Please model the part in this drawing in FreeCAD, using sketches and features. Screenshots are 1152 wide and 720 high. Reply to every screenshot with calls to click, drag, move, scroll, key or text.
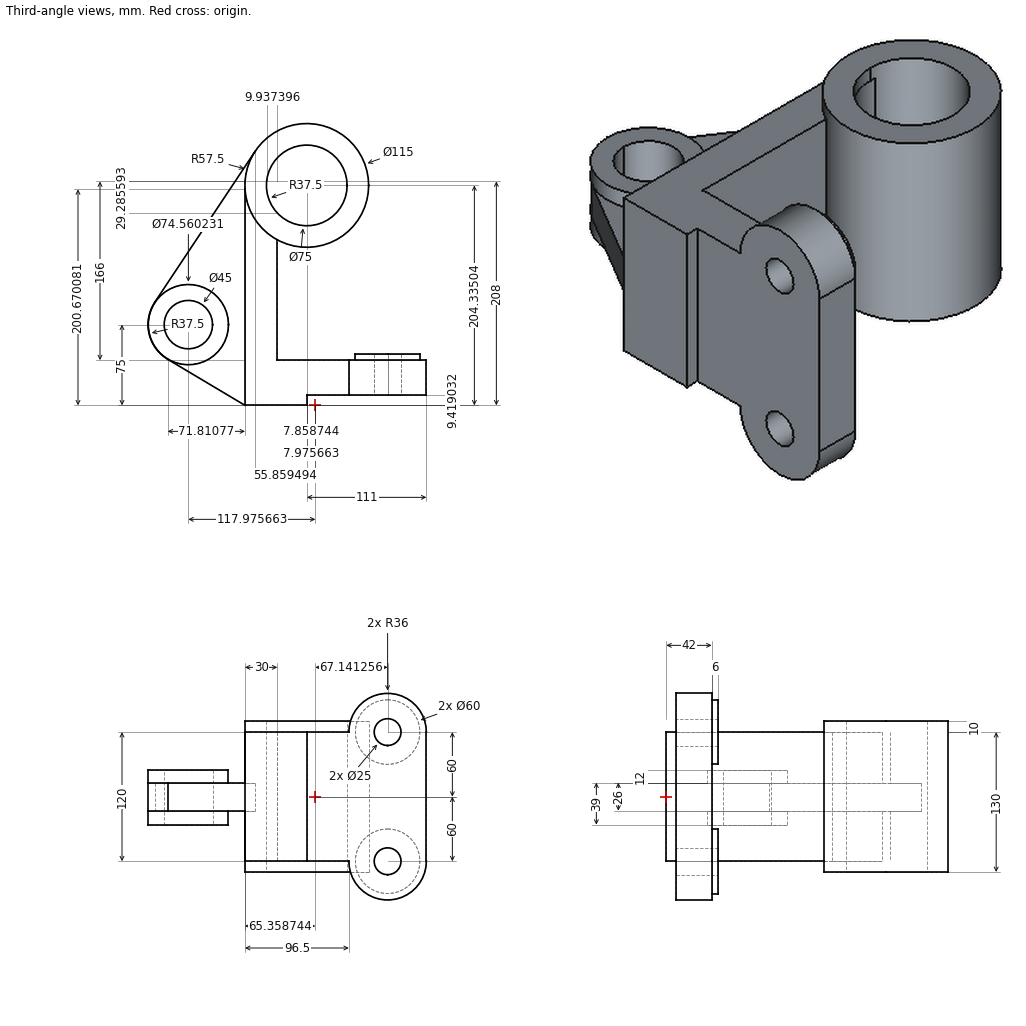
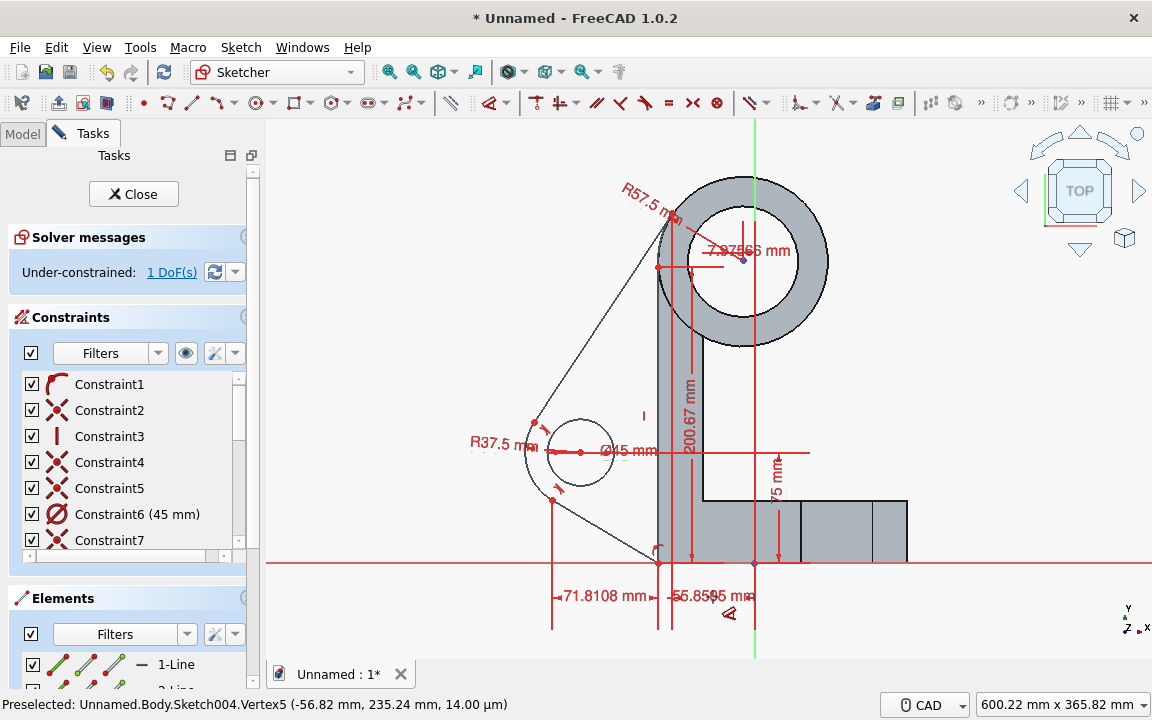
click(743, 261)
click(789, 412)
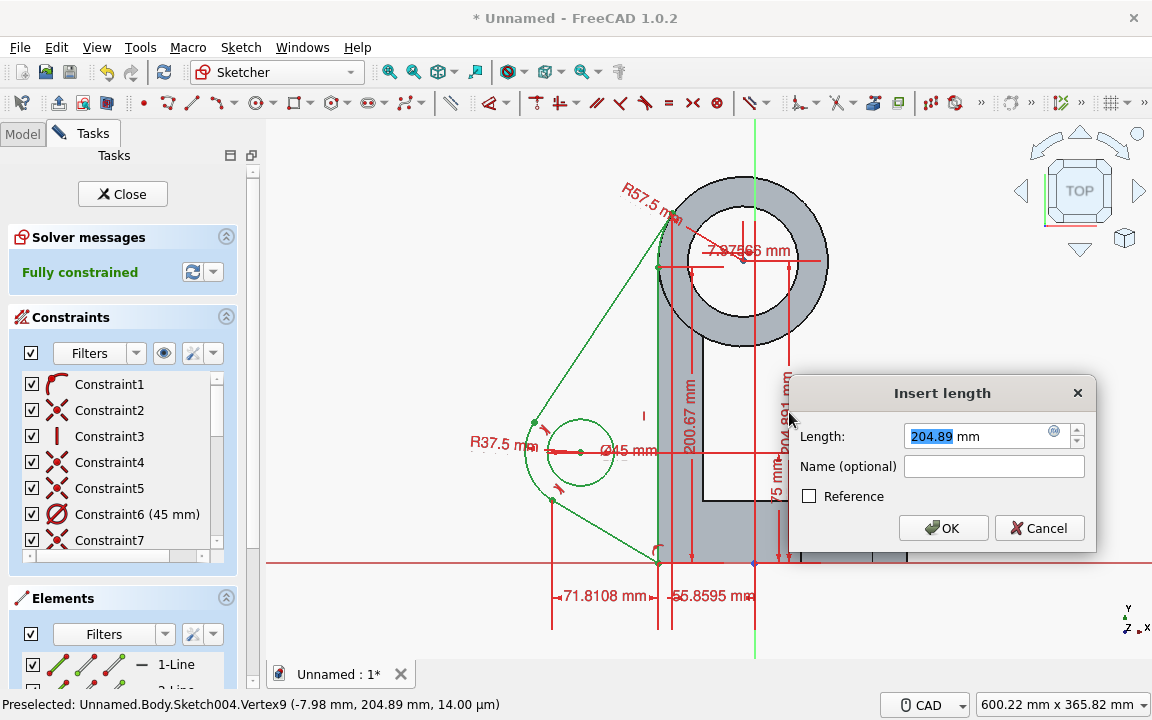
text(204.33504)
key(Return)
key(Escape)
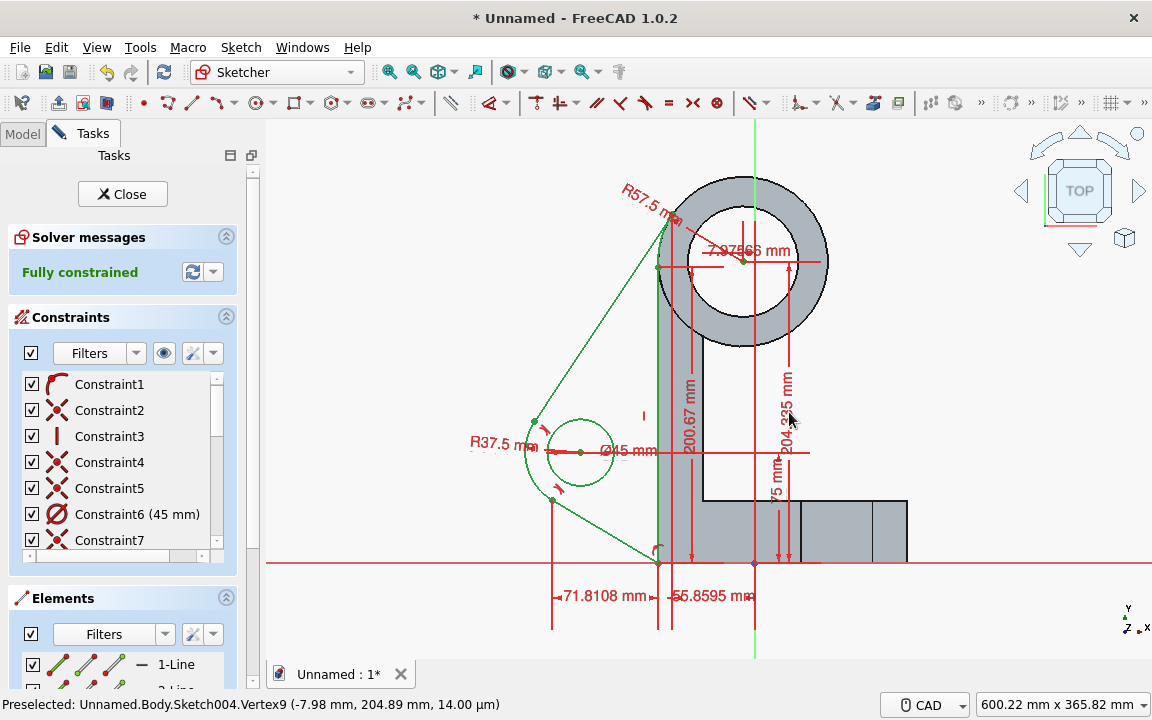
click(123, 194)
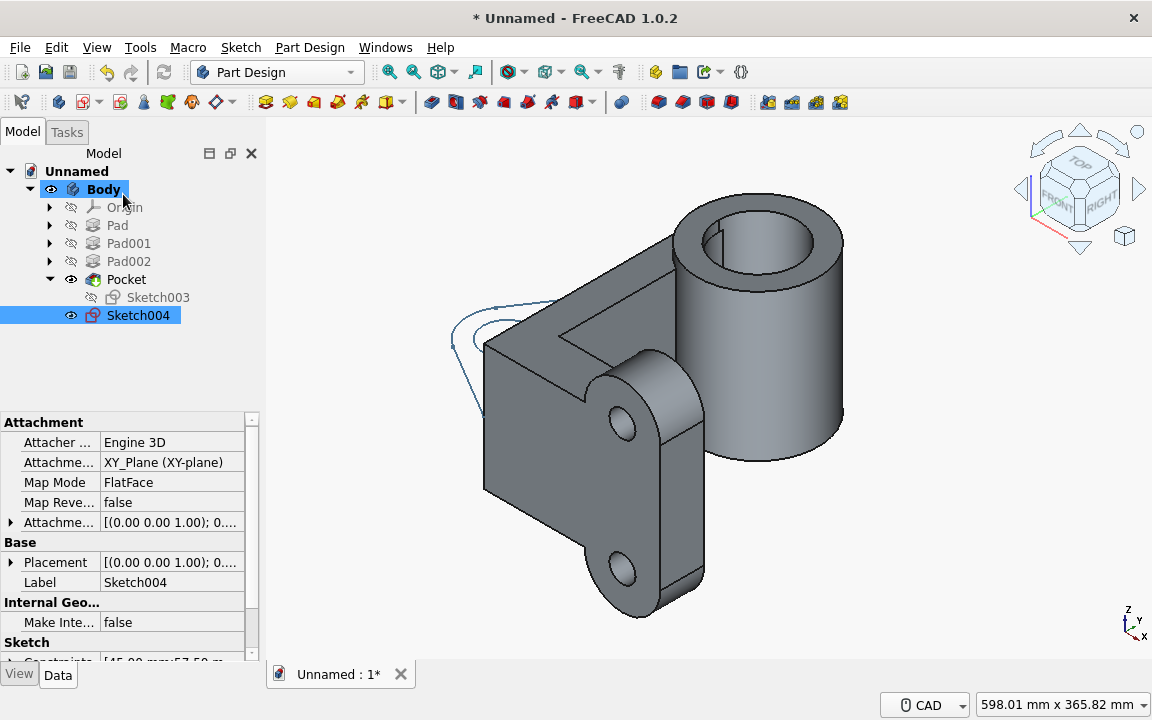
click(266, 102)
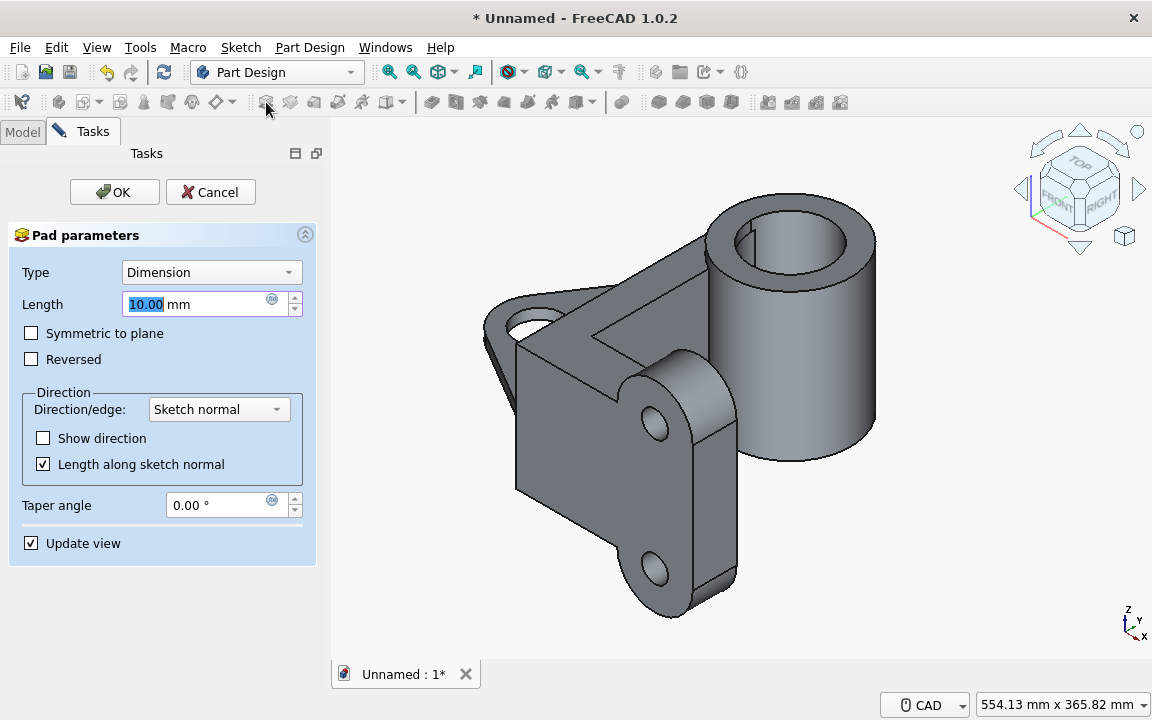
text(26)
key(Tab)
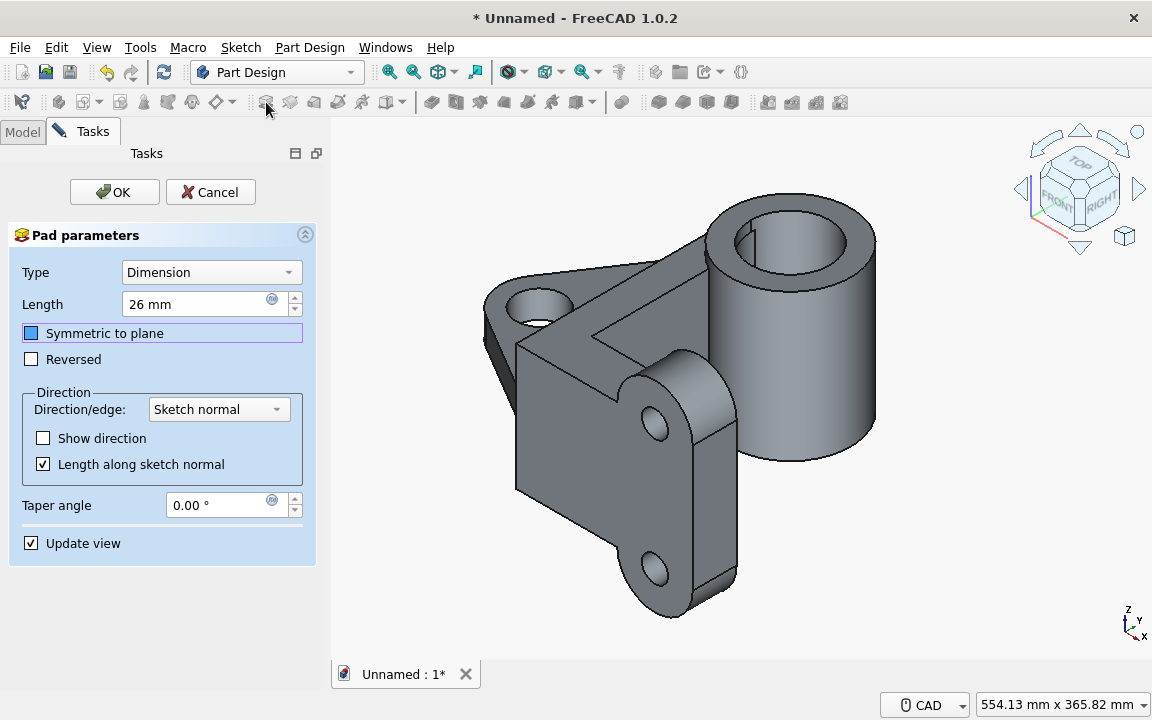
click(30, 333)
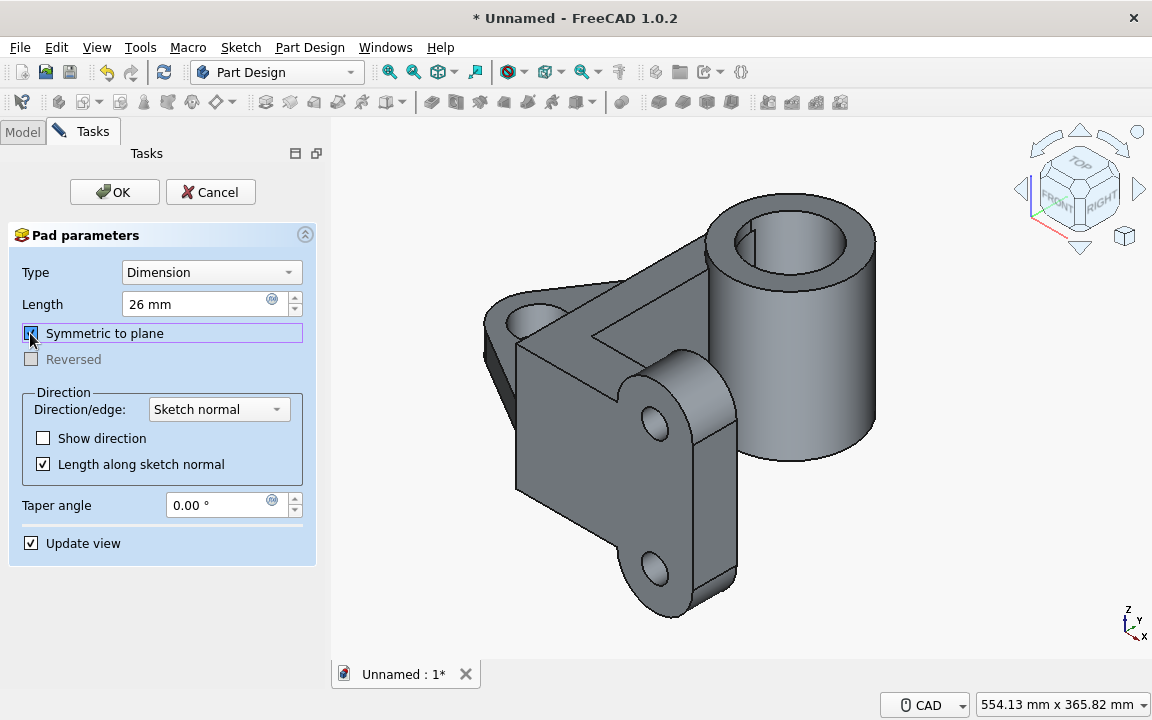
click(115, 192)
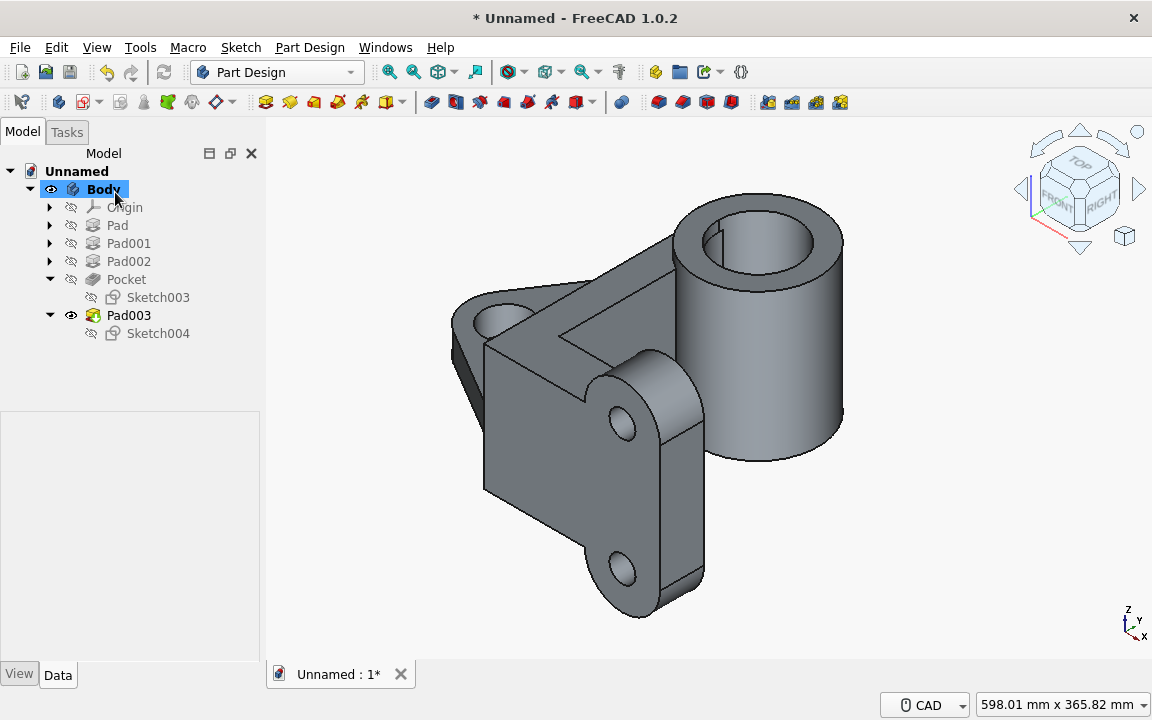
click(390, 72)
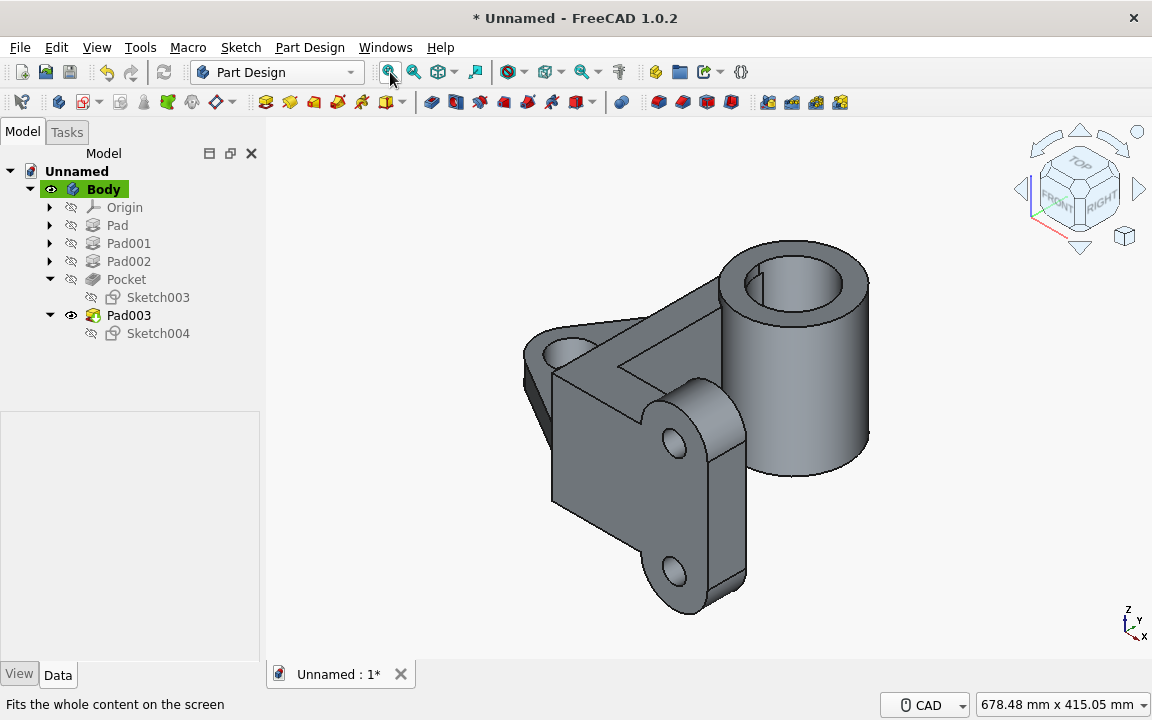
key(2)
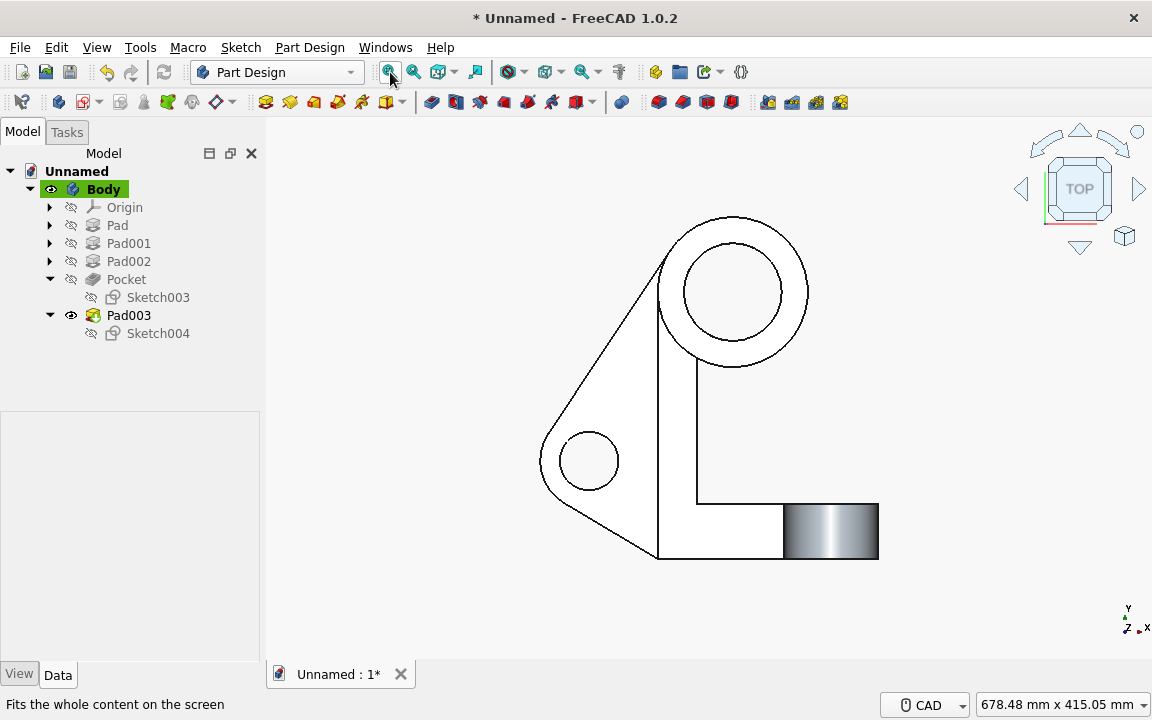
click(624, 404)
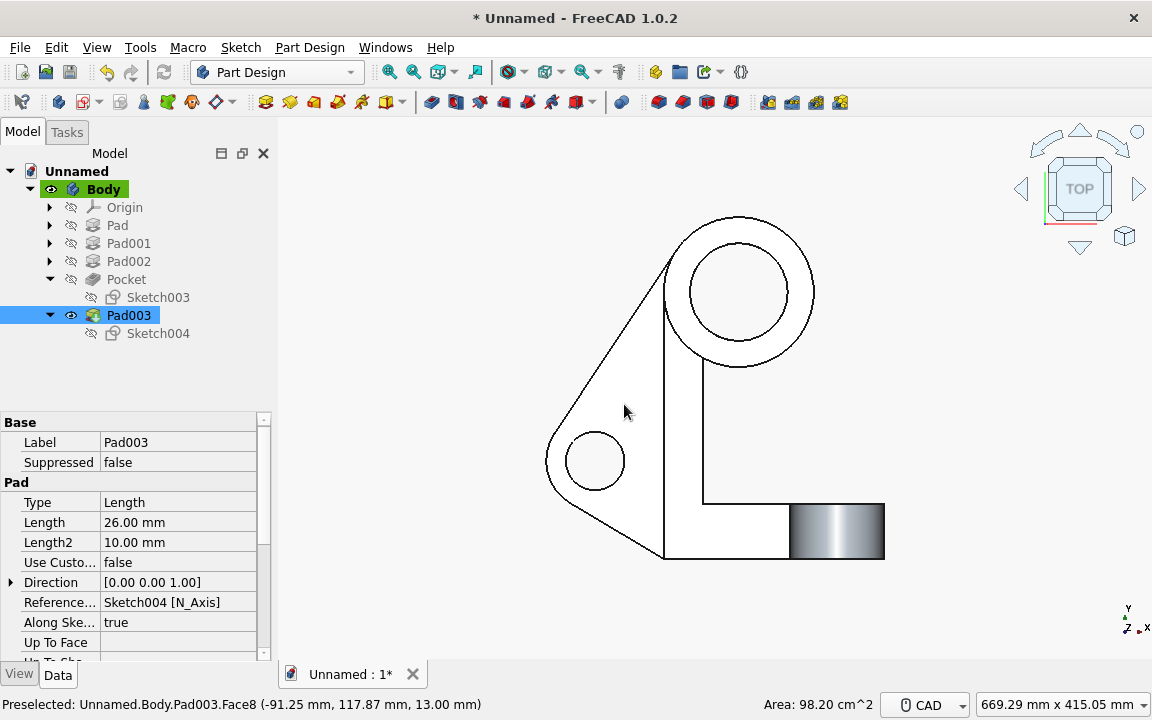
click(84, 102)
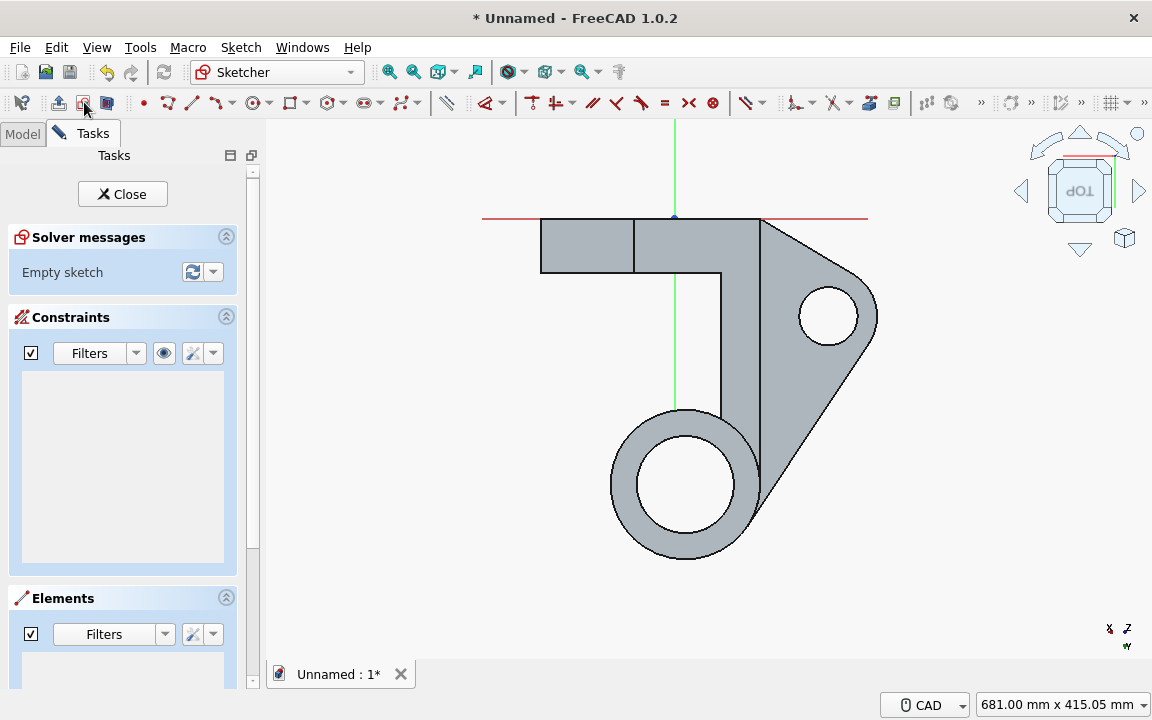
scroll(886, 212, up, 4)